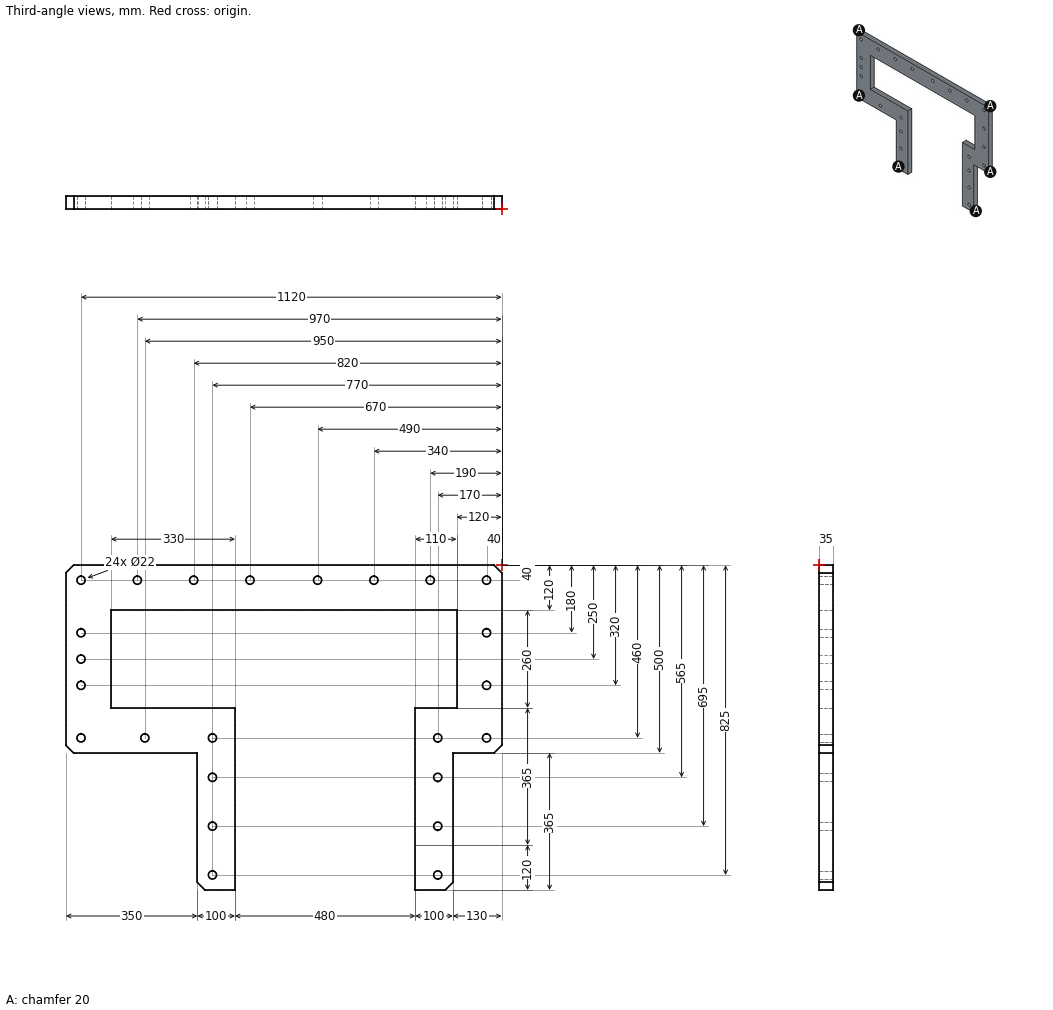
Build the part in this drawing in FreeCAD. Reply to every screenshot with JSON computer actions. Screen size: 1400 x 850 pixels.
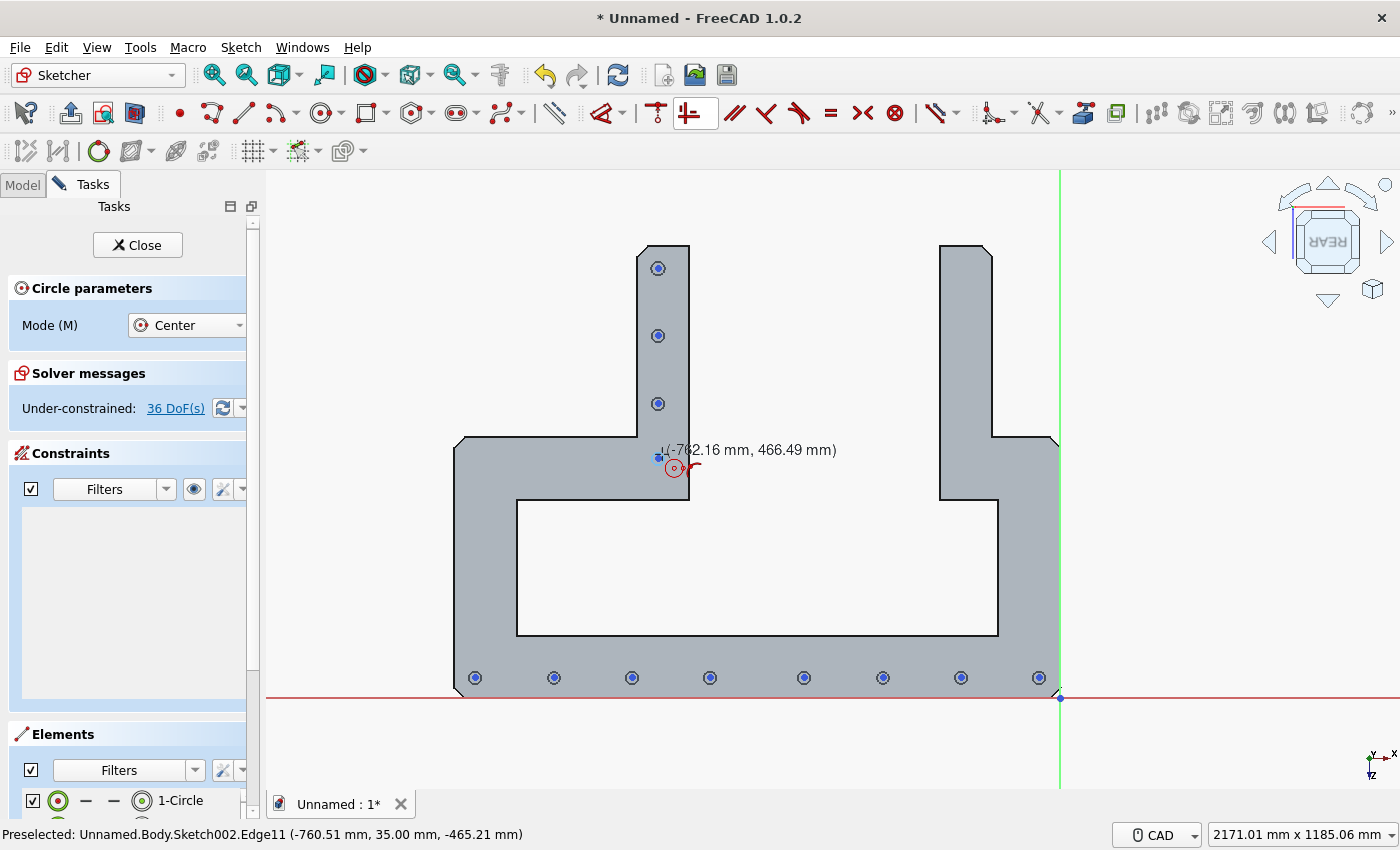
{"action": "scroll", "coordinate": [475, 604], "scroll_direction": "up", "scroll_amount": 7}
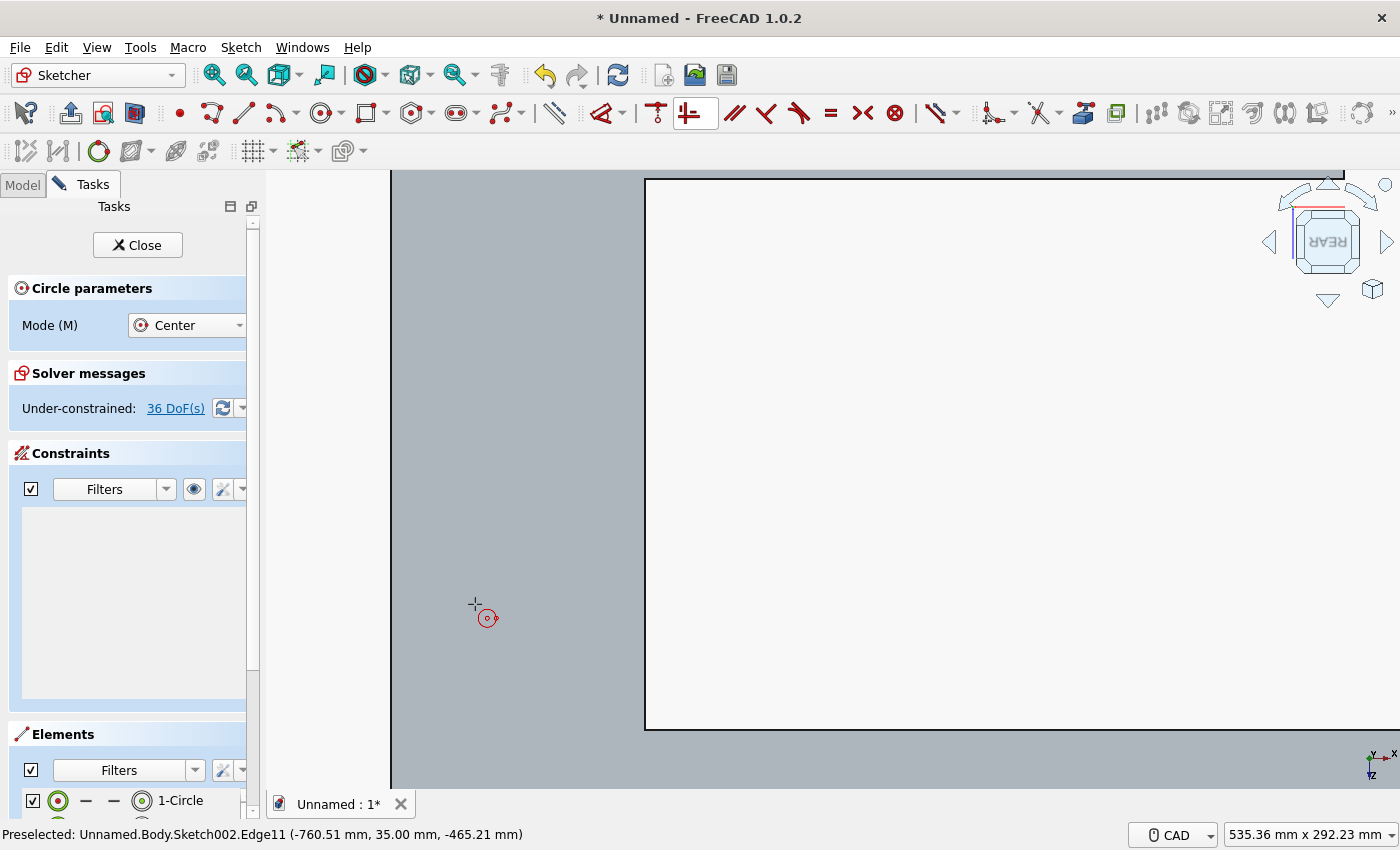
{"action": "scroll", "coordinate": [475, 604], "scroll_direction": "down", "scroll_amount": 7}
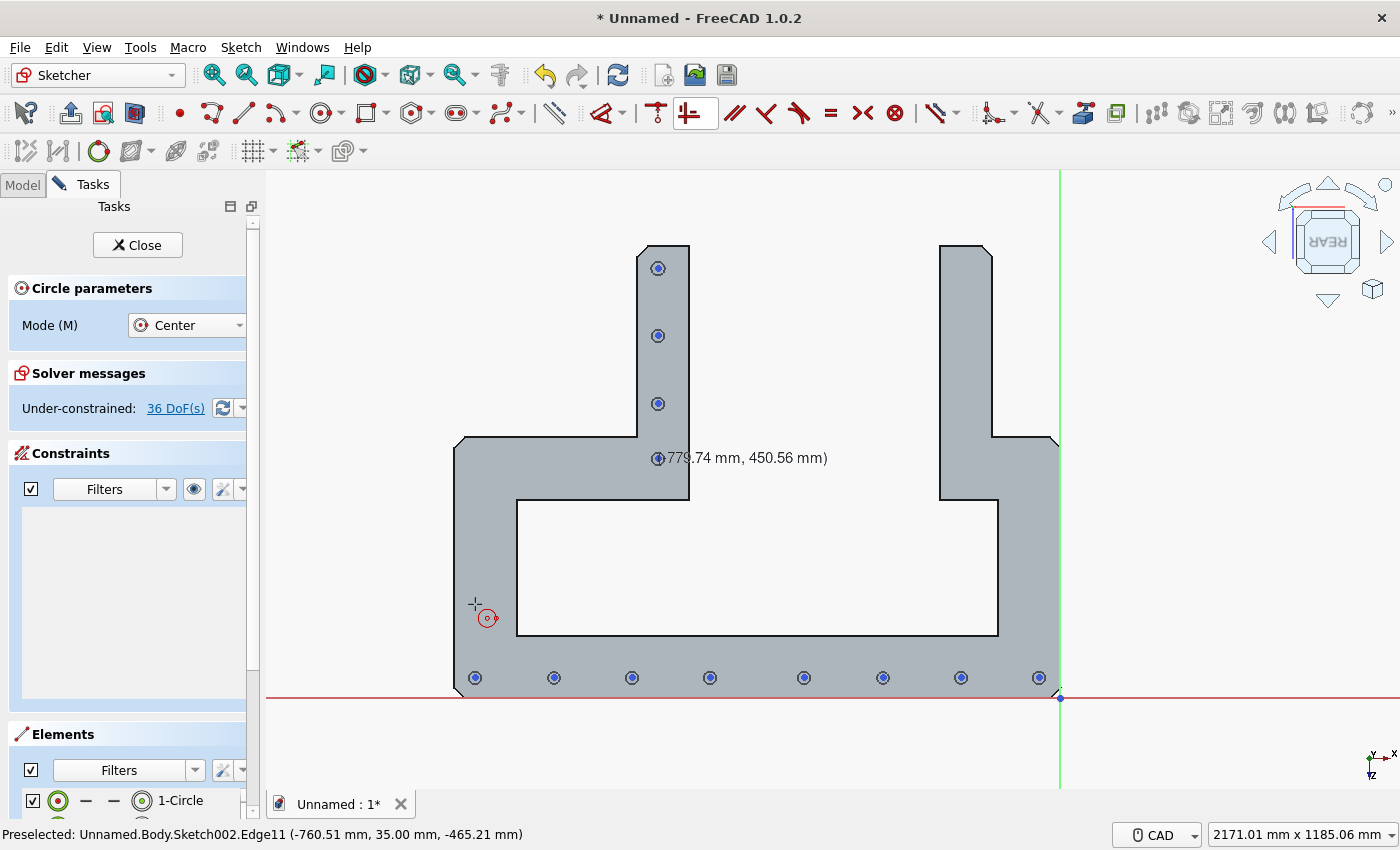
{"action": "left_click", "coordinate": [475, 604]}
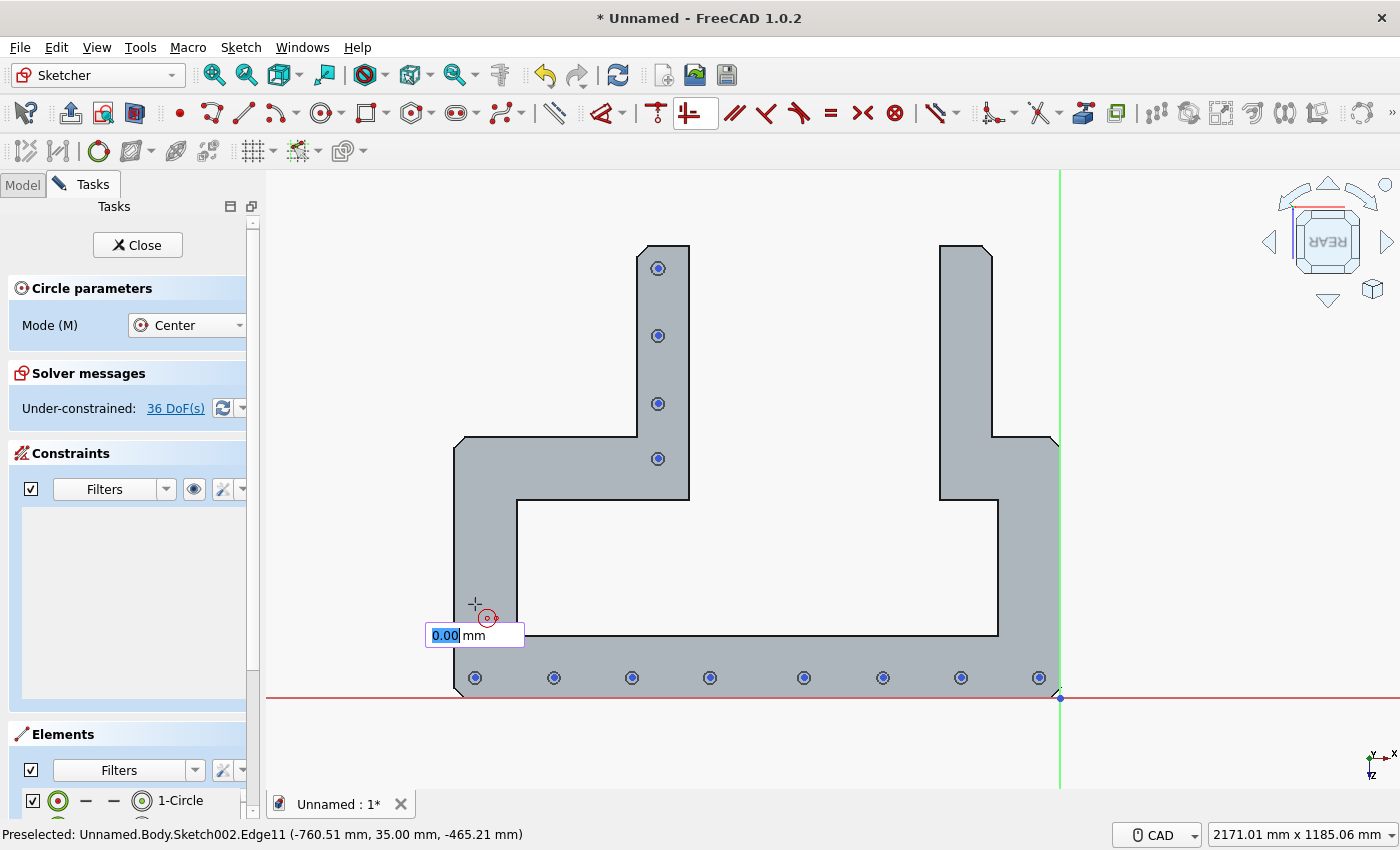
{"action": "scroll", "coordinate": [479, 600], "scroll_direction": "up", "scroll_amount": 6}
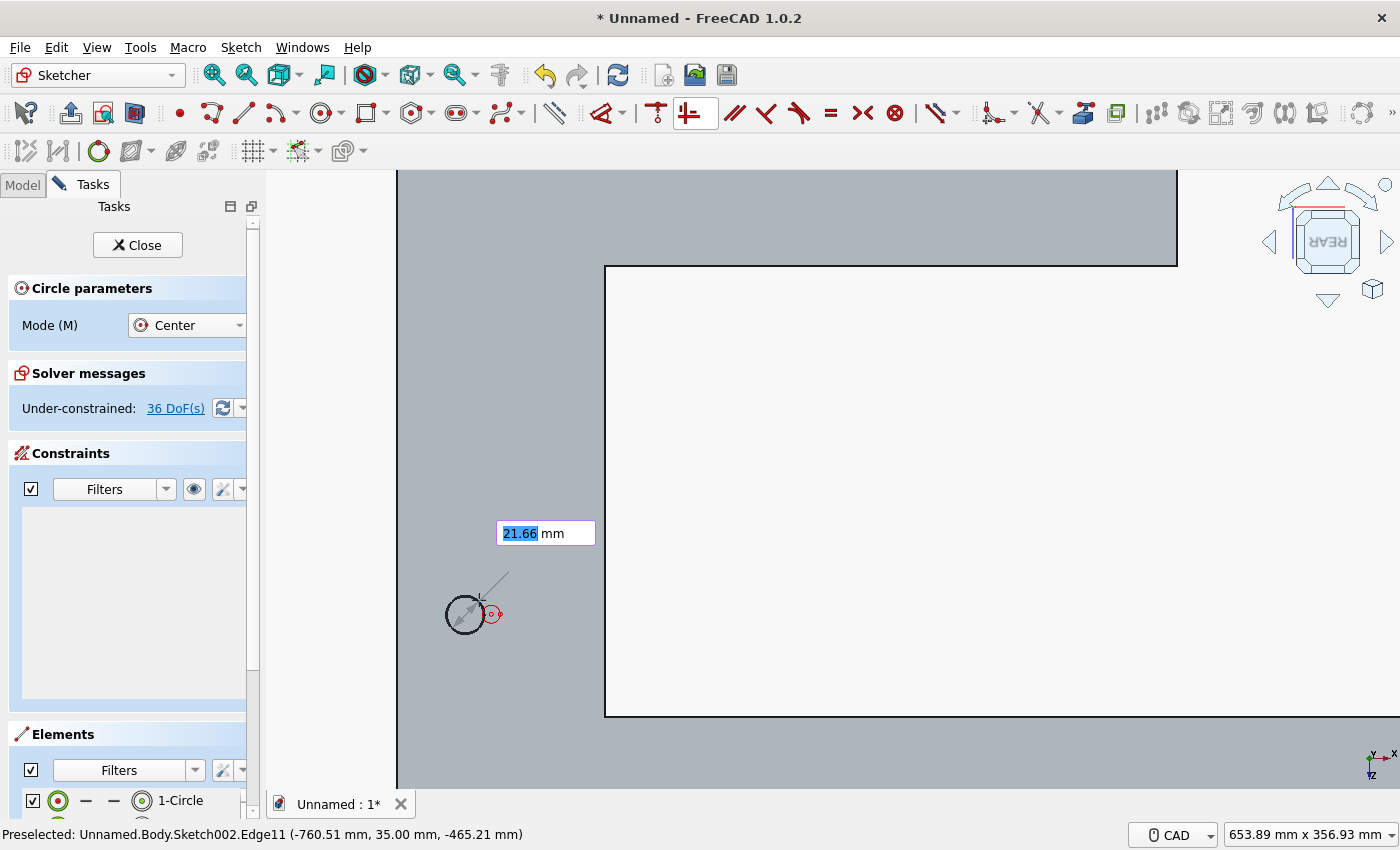
{"action": "left_click", "coordinate": [480, 599]}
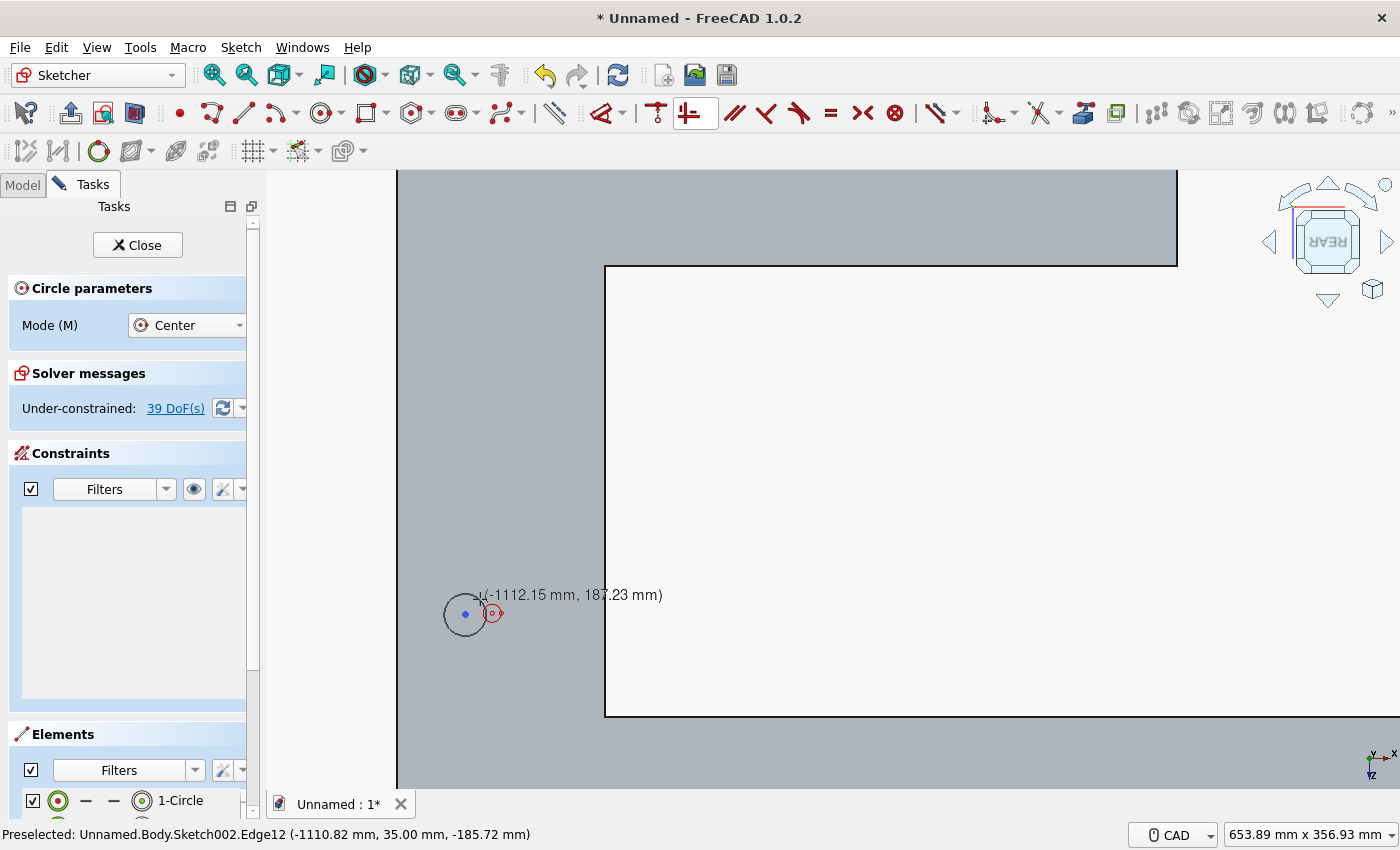
{"action": "scroll", "coordinate": [479, 600], "scroll_direction": "down", "scroll_amount": 6}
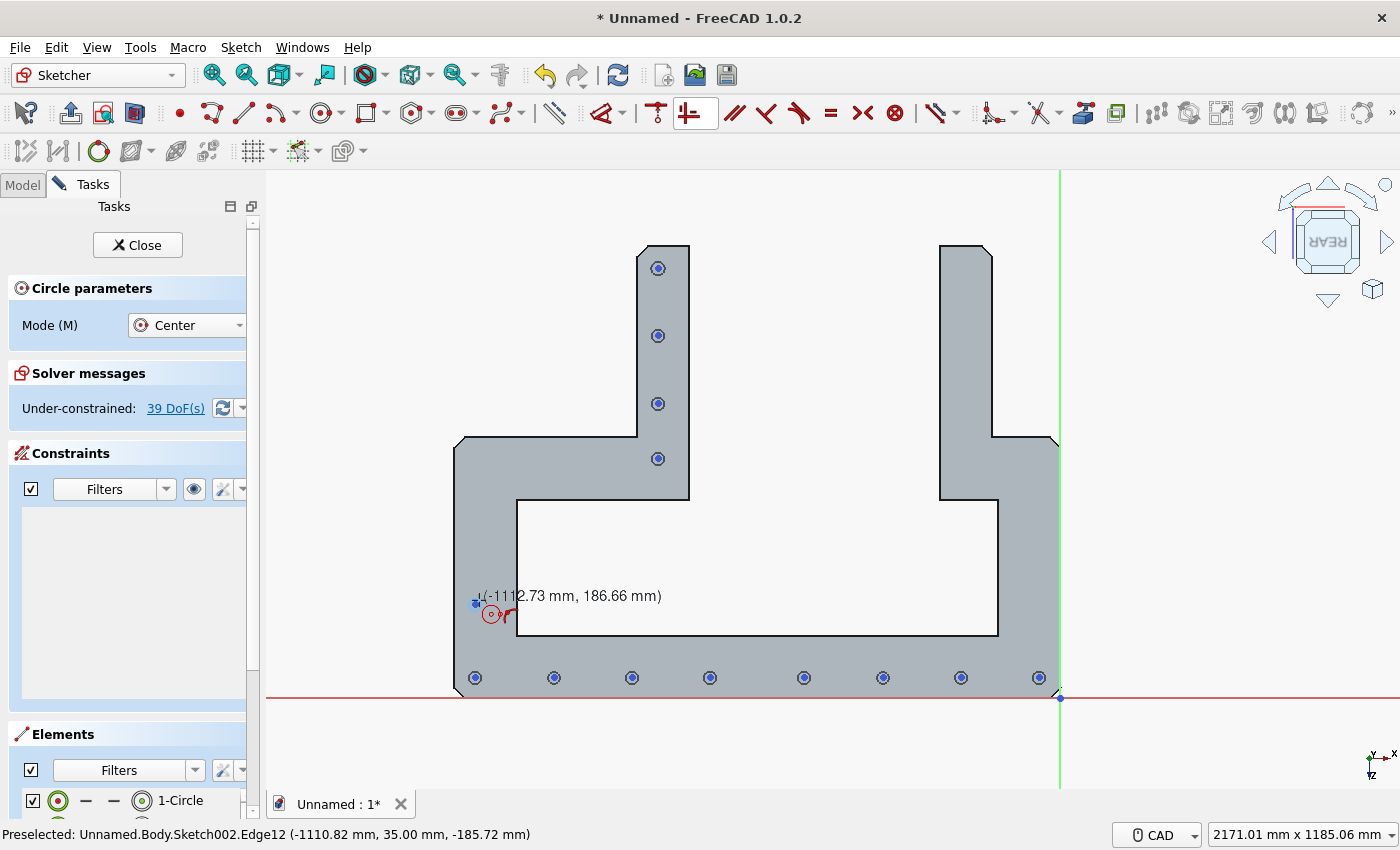
{"action": "left_click", "coordinate": [475, 568]}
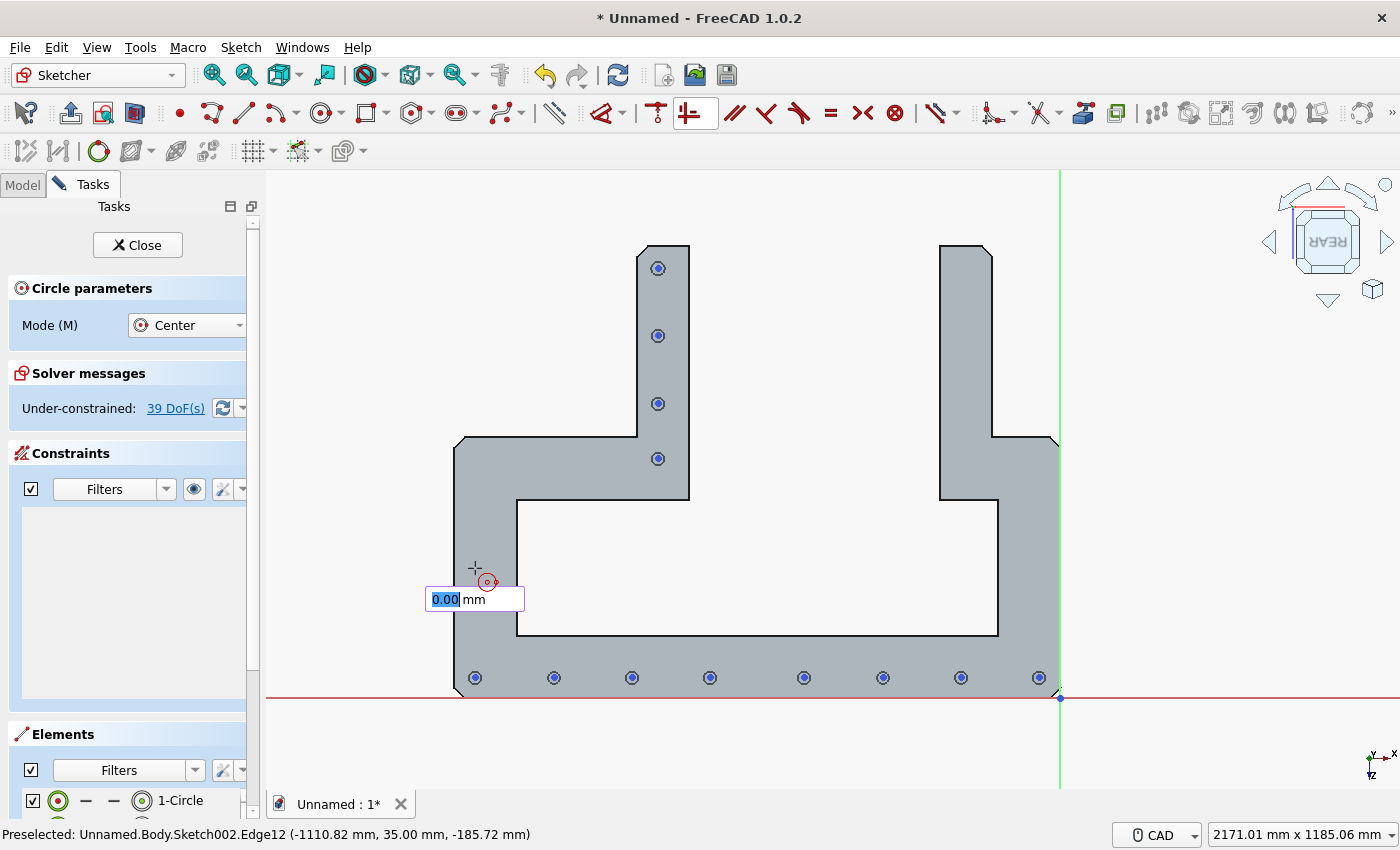
{"action": "scroll", "coordinate": [479, 564], "scroll_direction": "up", "scroll_amount": 6}